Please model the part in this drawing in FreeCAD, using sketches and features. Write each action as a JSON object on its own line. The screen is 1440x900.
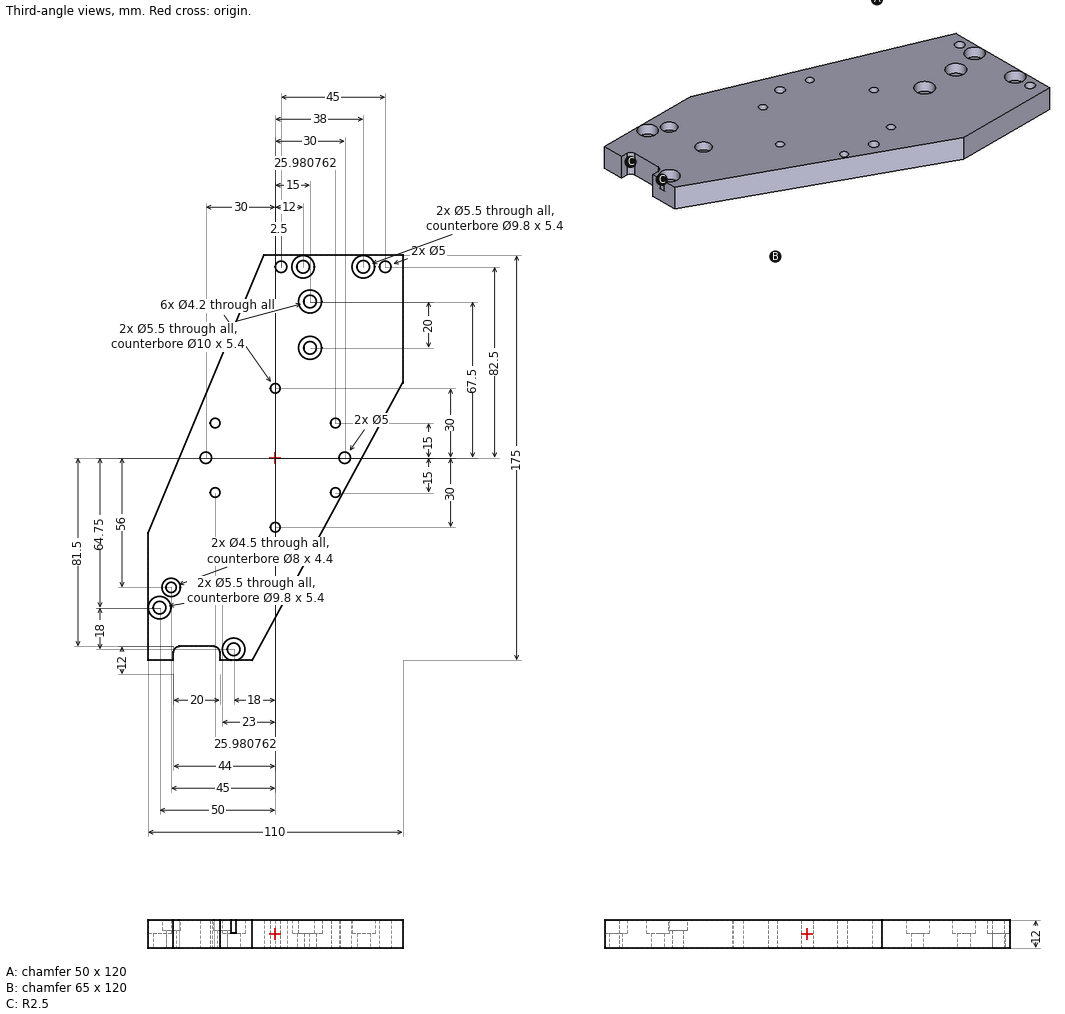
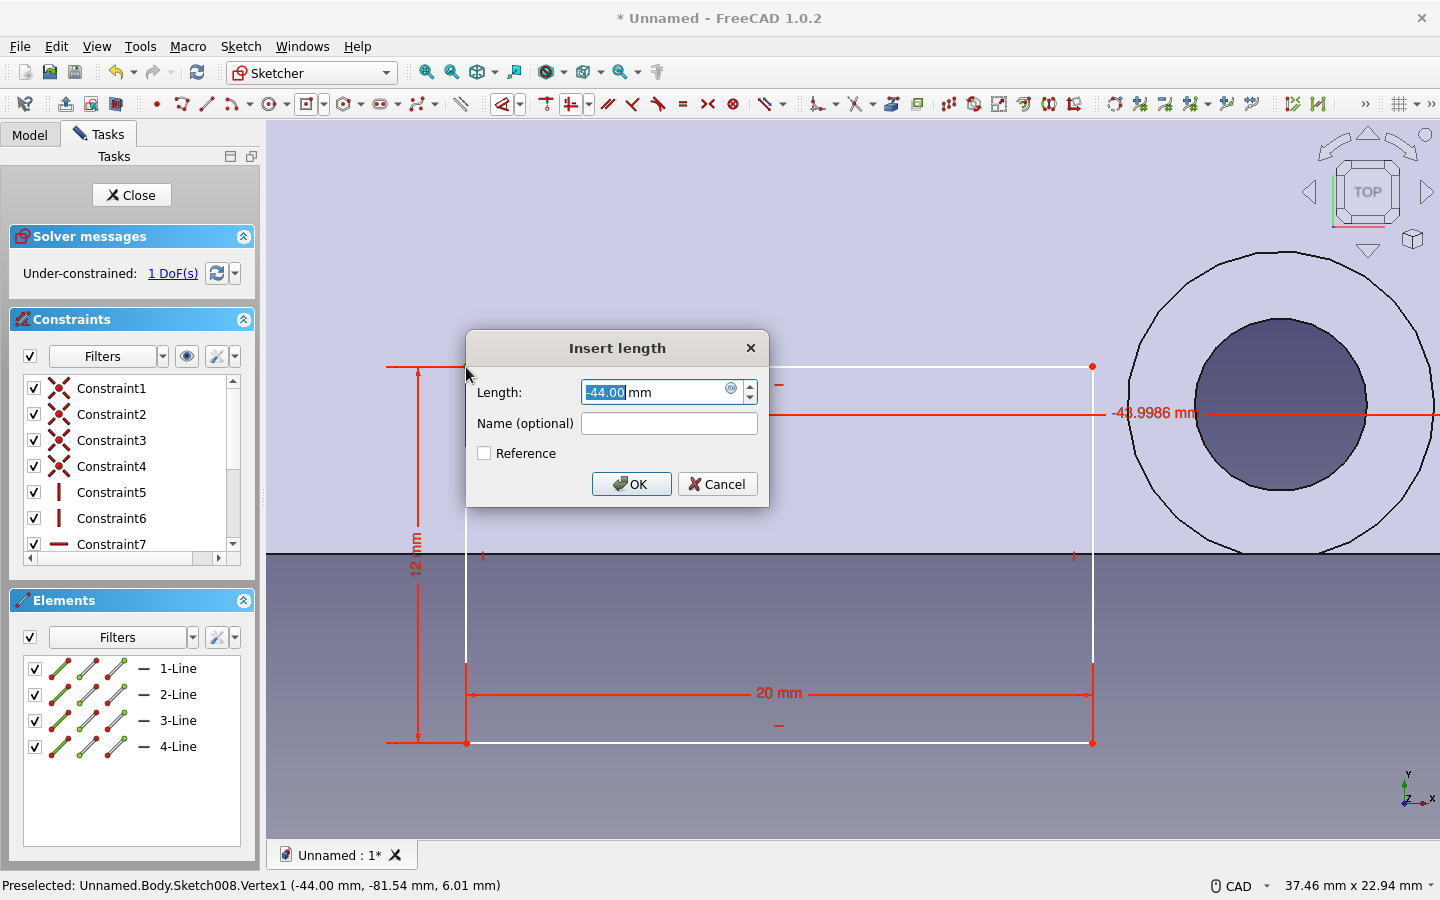
{"action": "type", "text": "-44"}
{"action": "key", "text": "Return"}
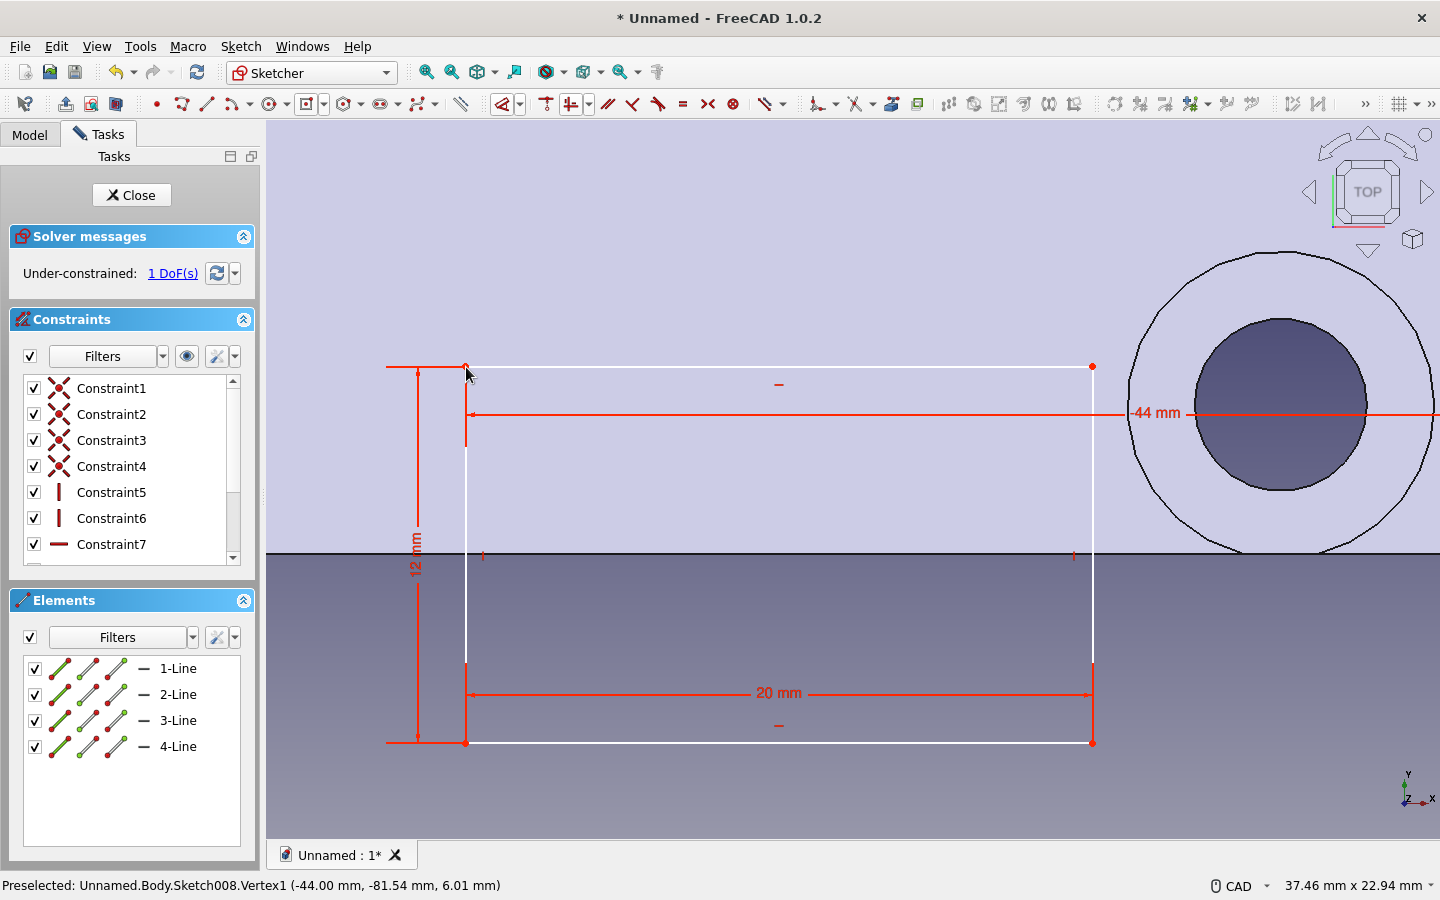
{"action": "left_click", "coordinate": [466, 367]}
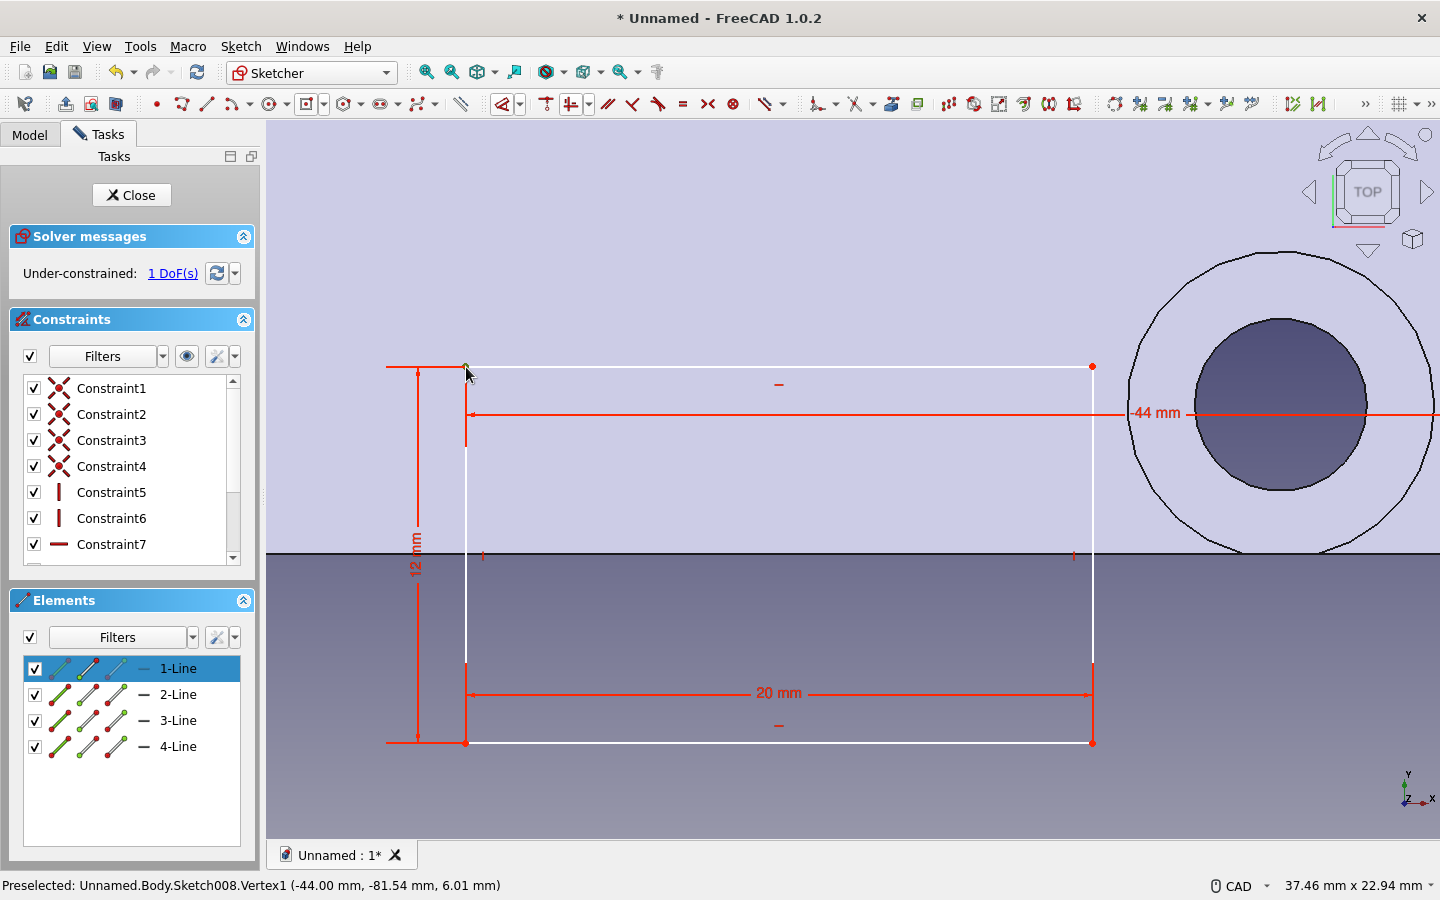
{"action": "key", "text": "i"}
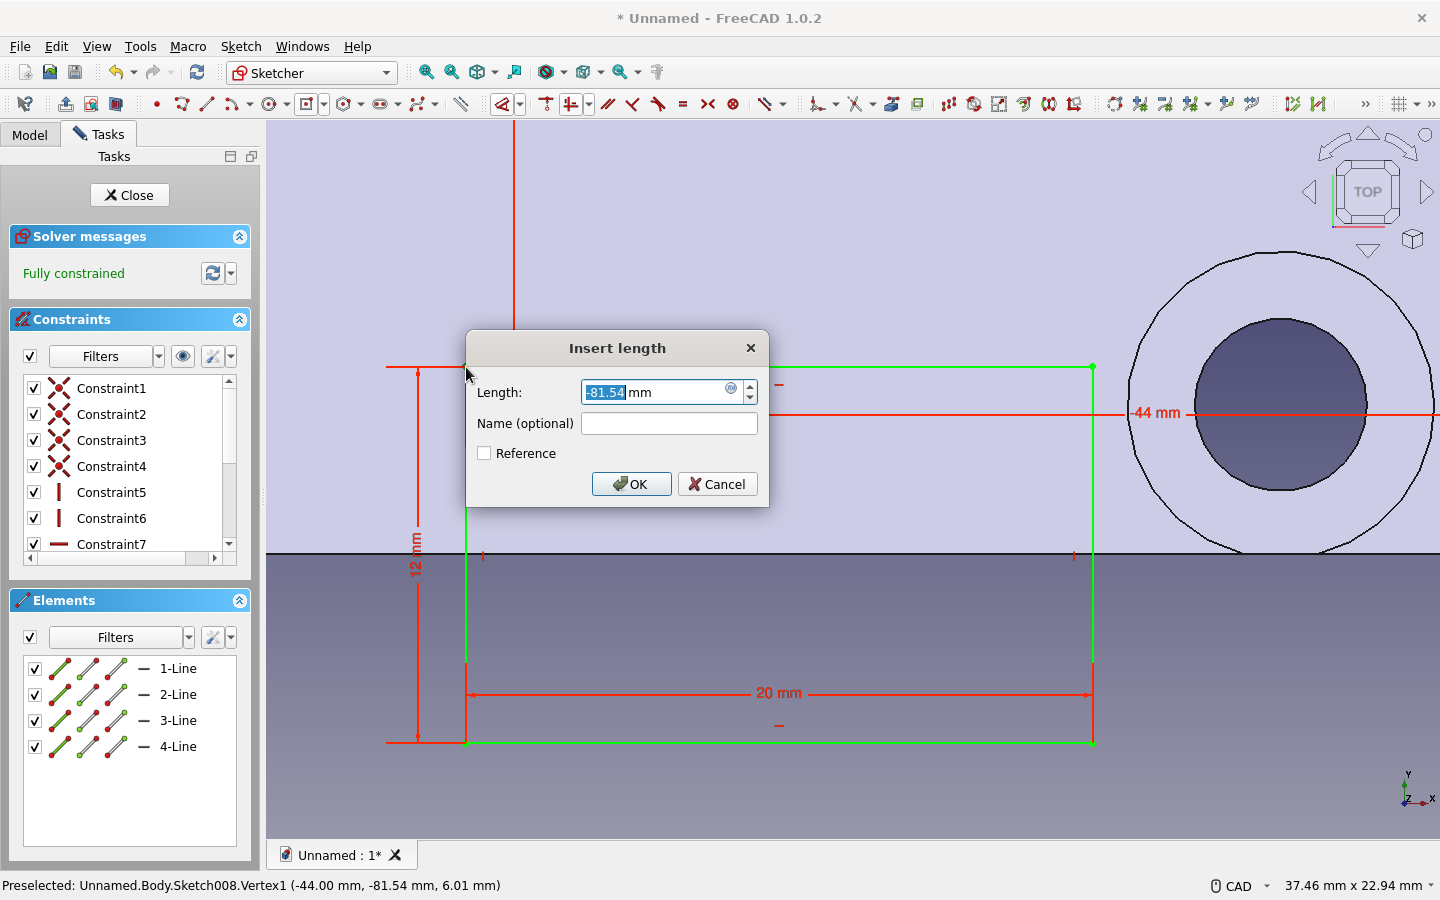
{"action": "type", "text": "-81.5"}
{"action": "key", "text": "Return"}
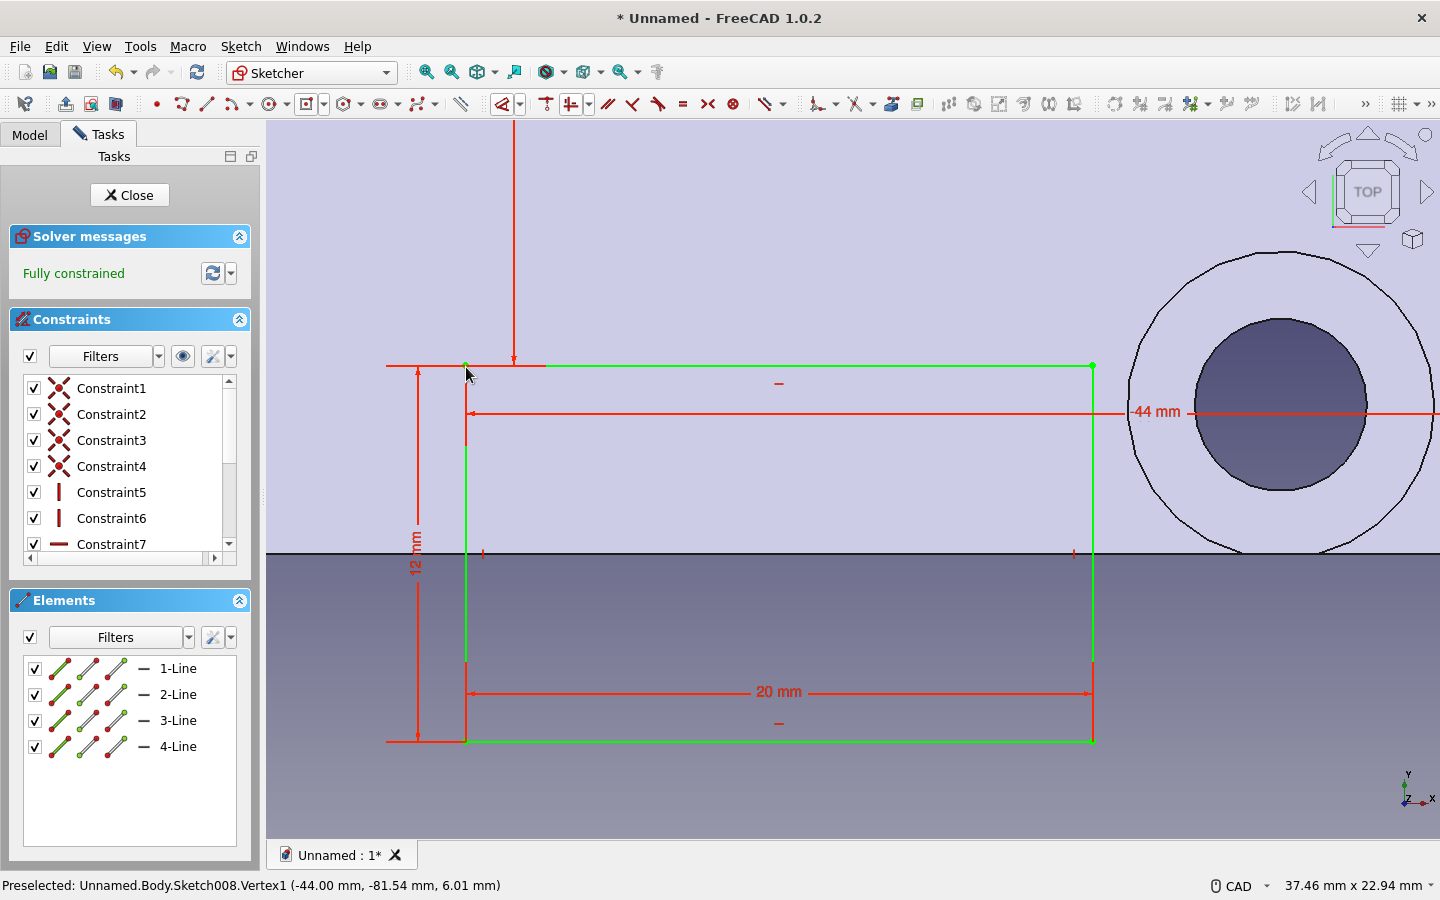
{"action": "left_click", "coordinate": [130, 195]}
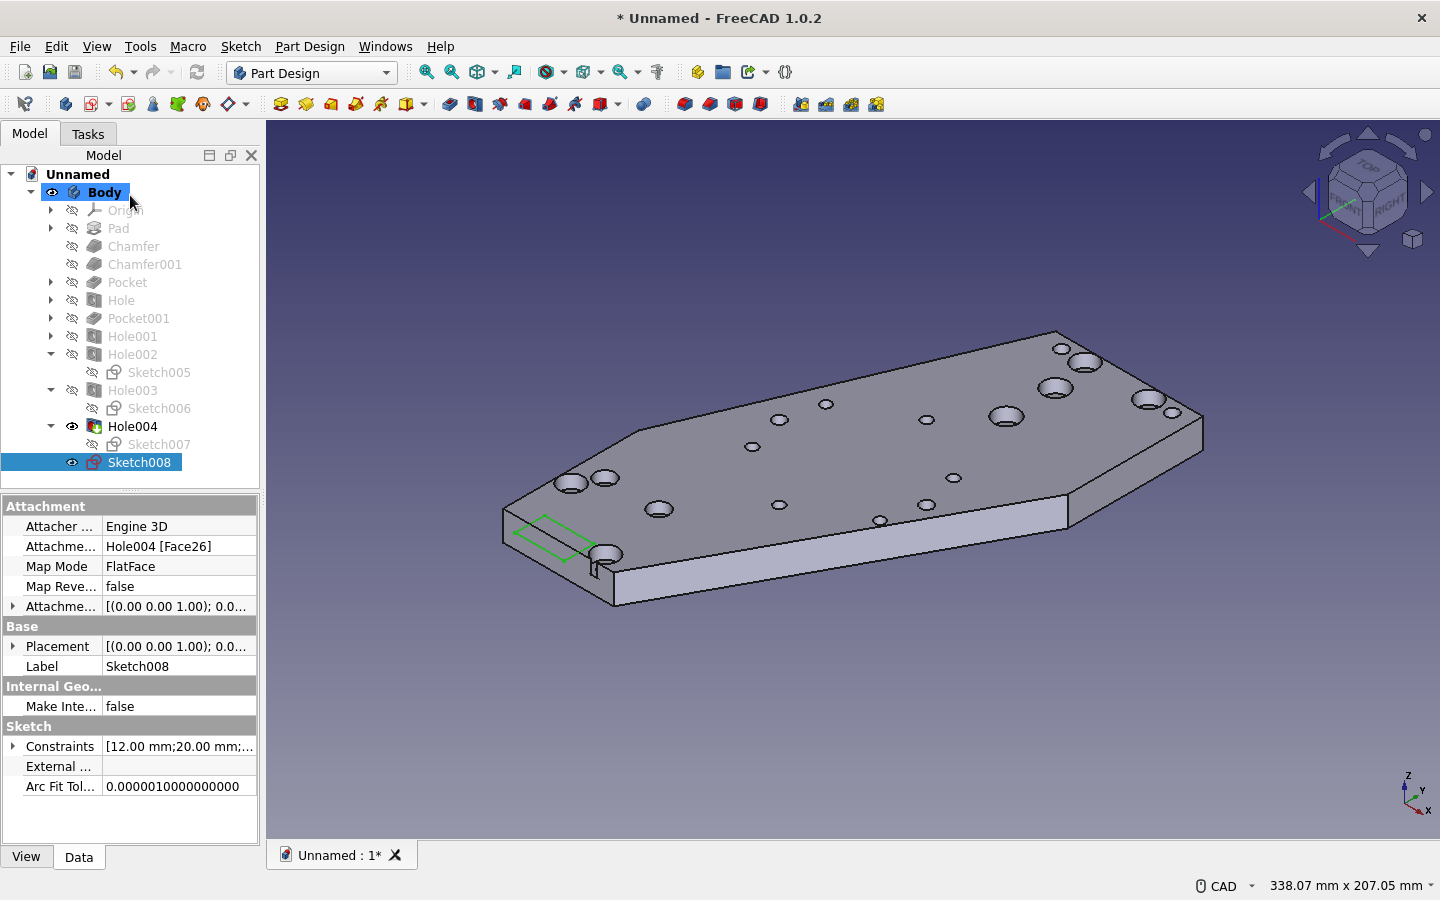
{"action": "left_click", "coordinate": [450, 104]}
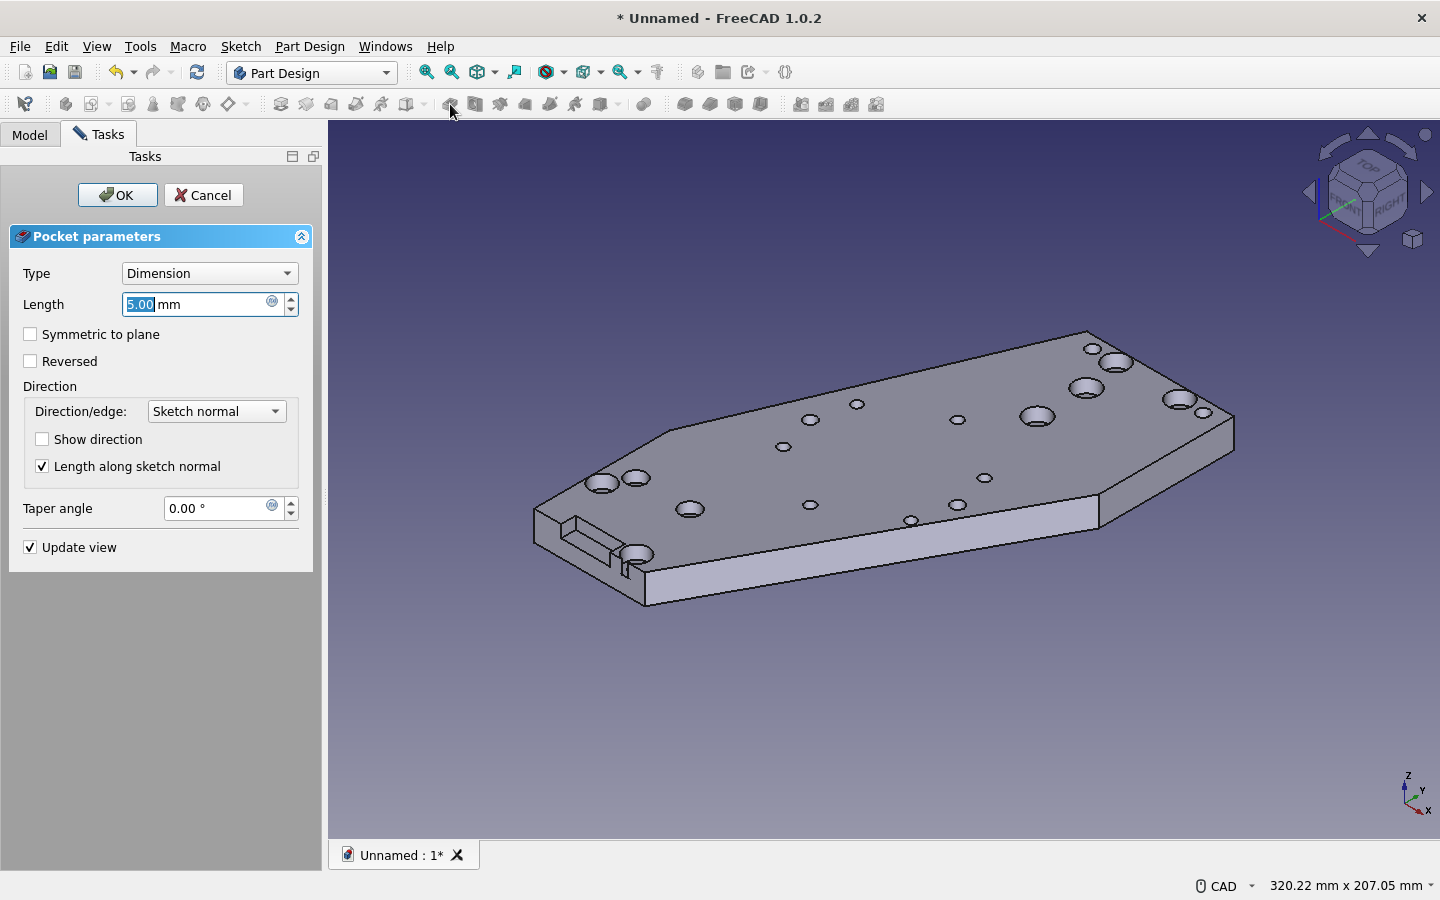
{"action": "left_click", "coordinate": [210, 274]}